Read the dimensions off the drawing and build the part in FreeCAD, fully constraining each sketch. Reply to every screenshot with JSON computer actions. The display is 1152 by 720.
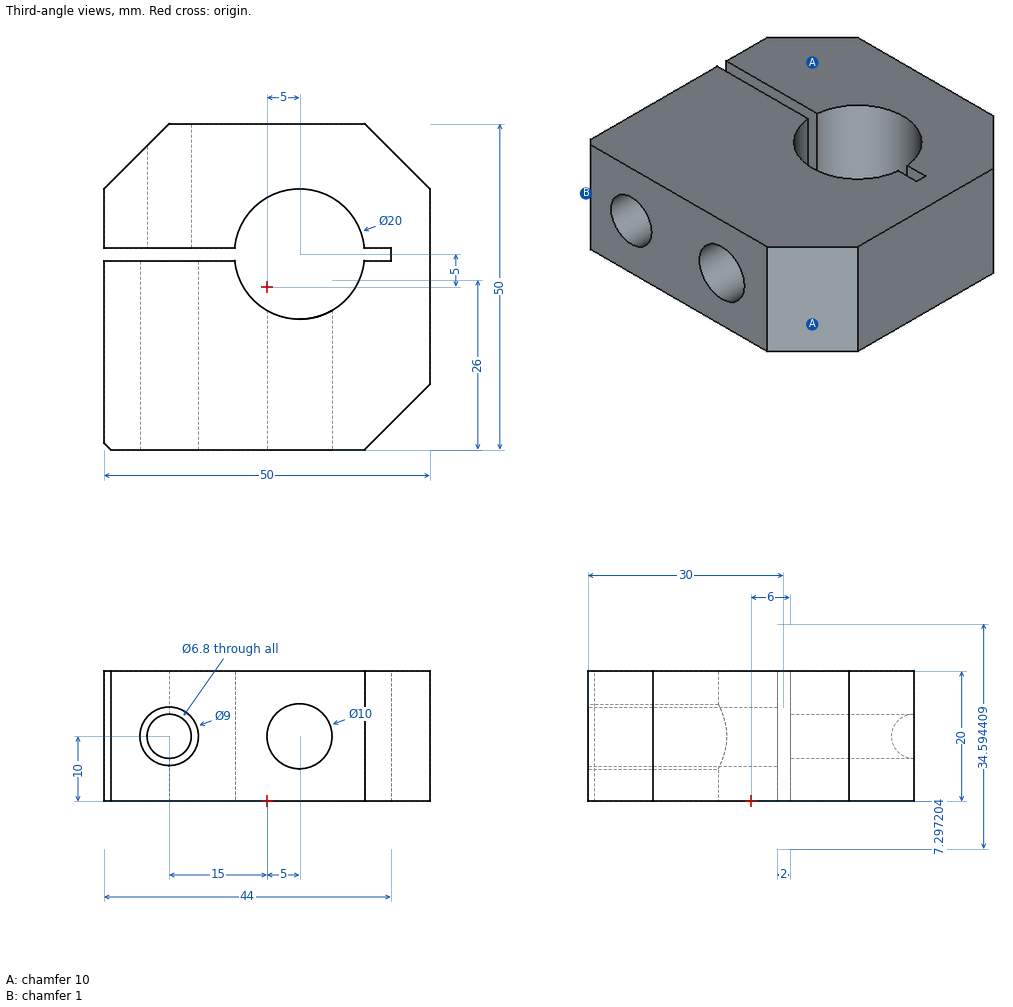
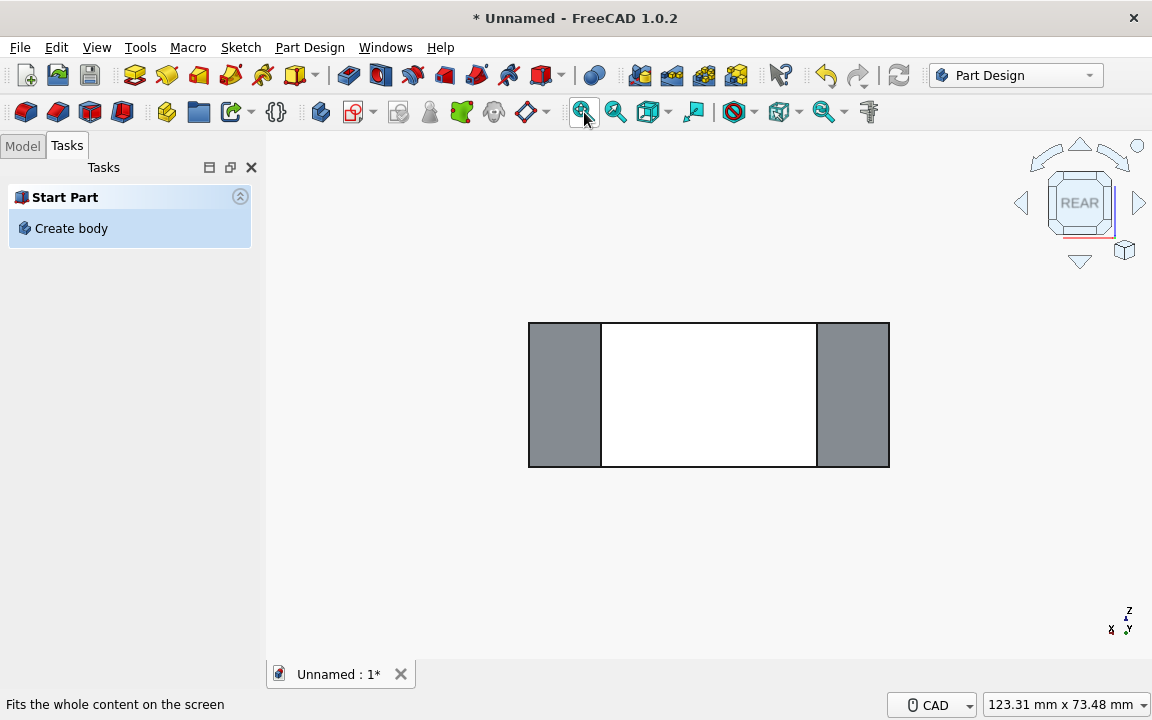
{"action": "key", "text": "0"}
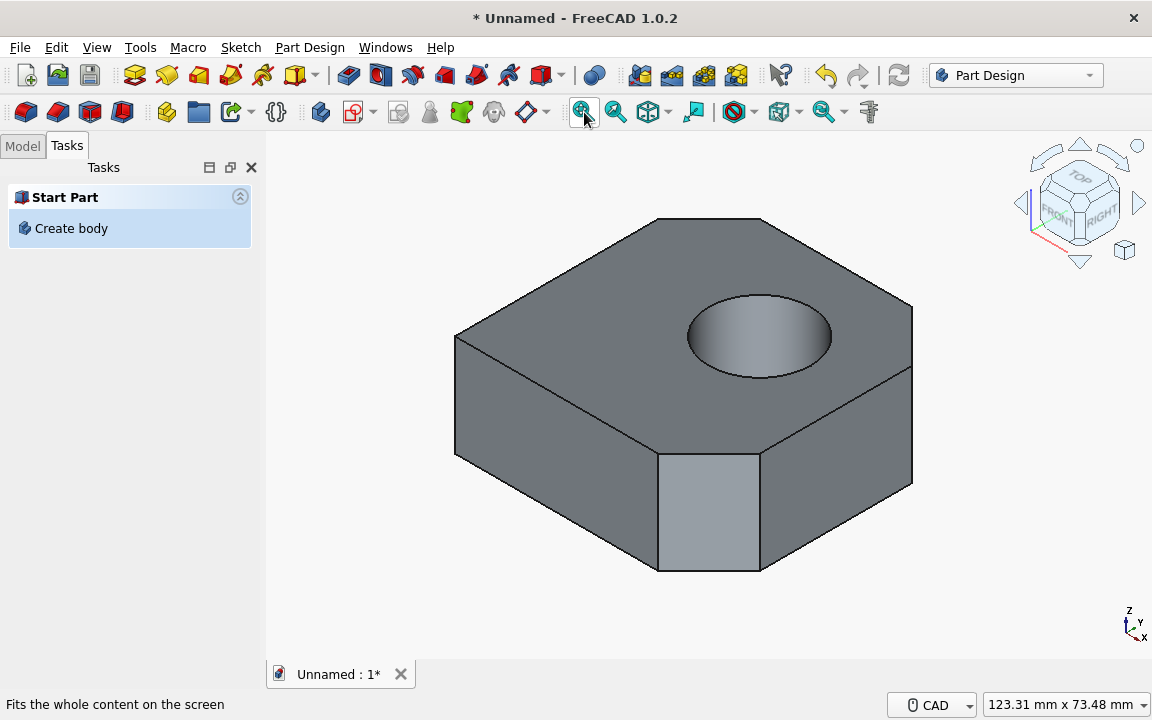
{"action": "key", "text": "2"}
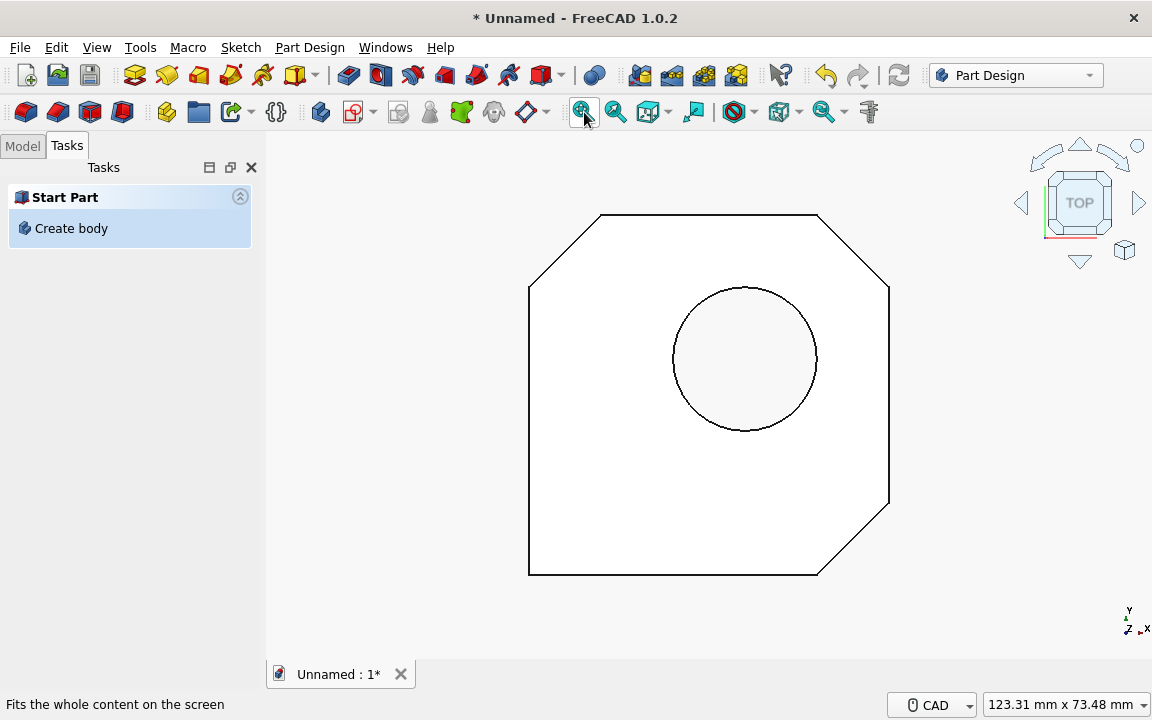
{"action": "key", "text": "1"}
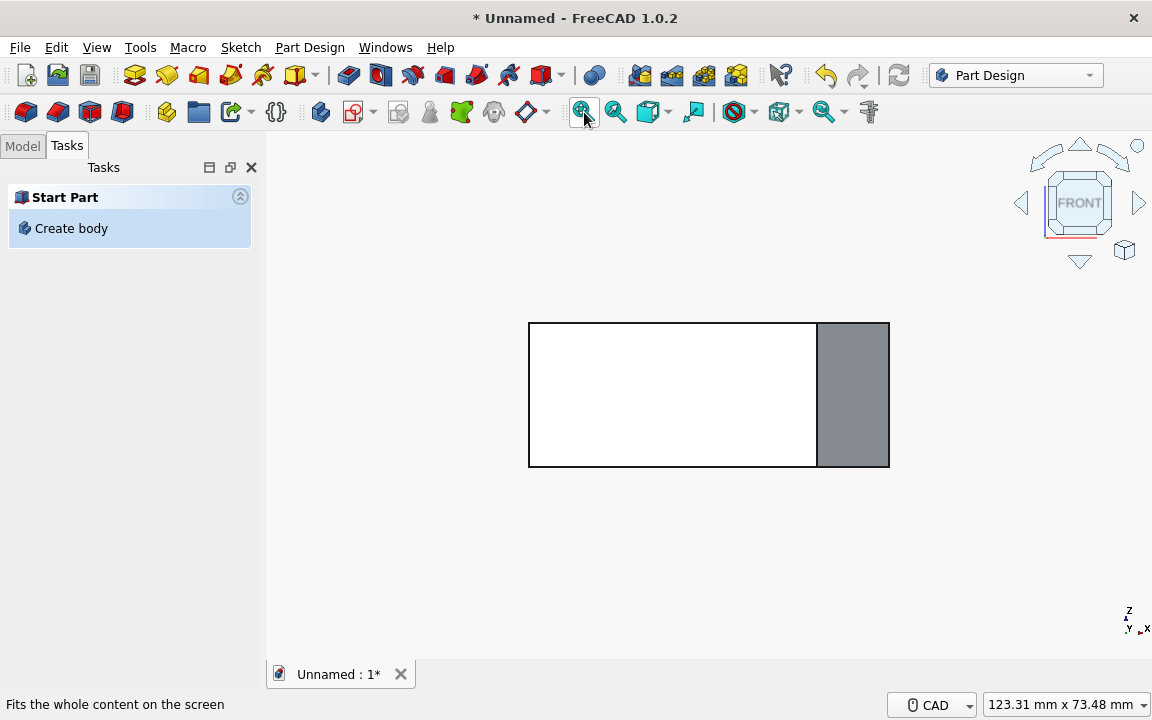
{"action": "left_click", "coordinate": [584, 112]}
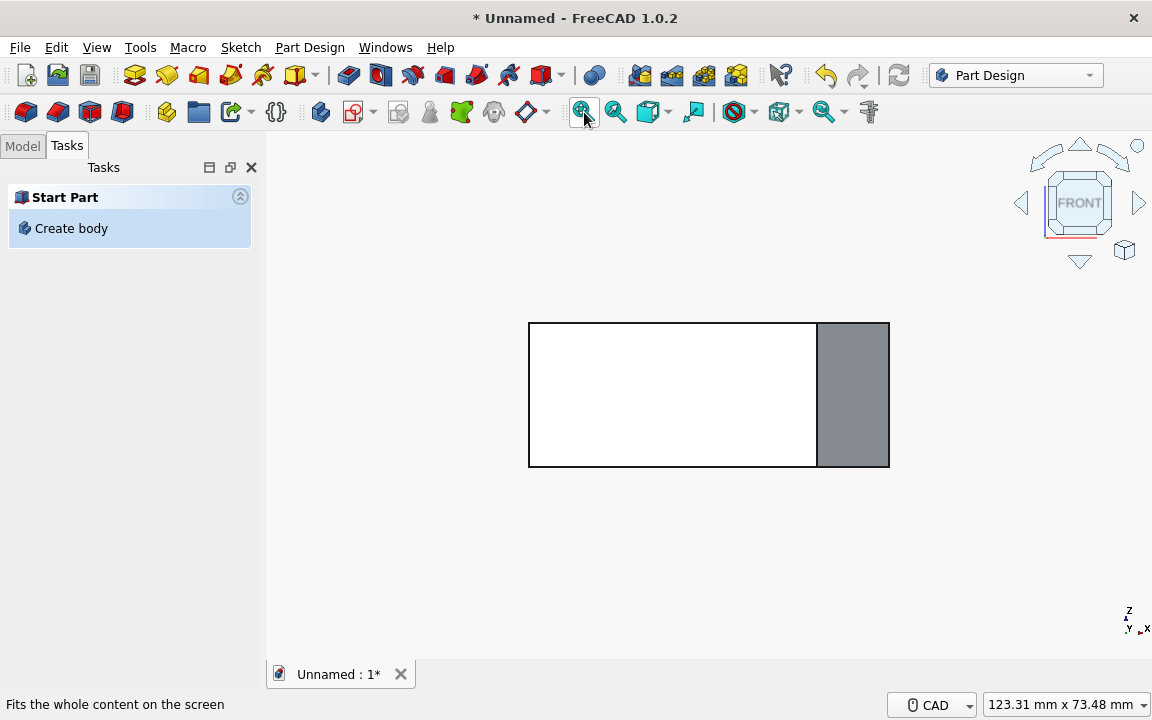
{"action": "left_click", "coordinate": [529, 394]}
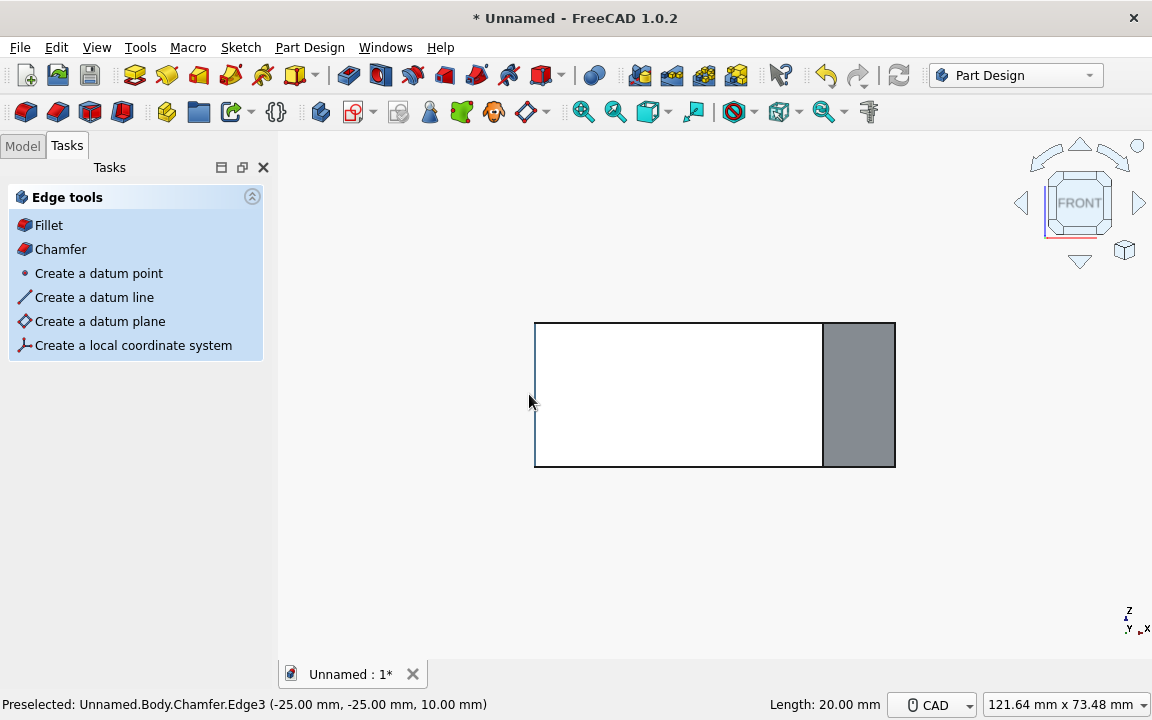
{"action": "left_click", "coordinate": [58, 112]}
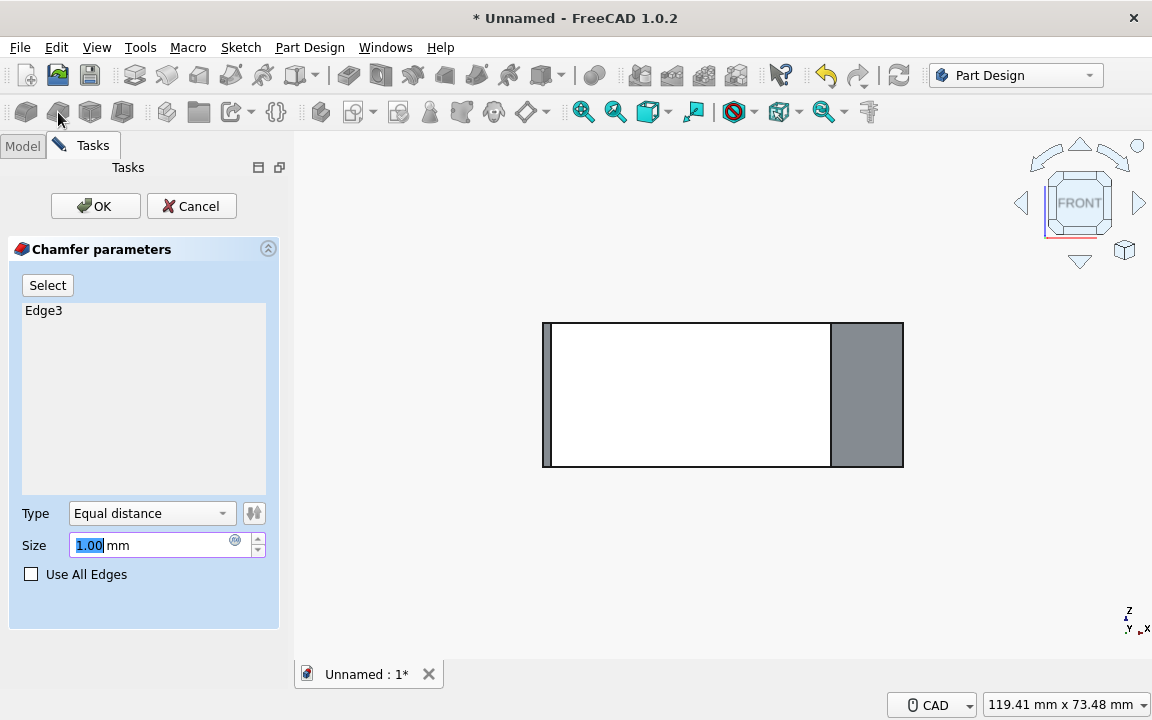
{"action": "type", "text": "1"}
{"action": "key", "text": "Tab"}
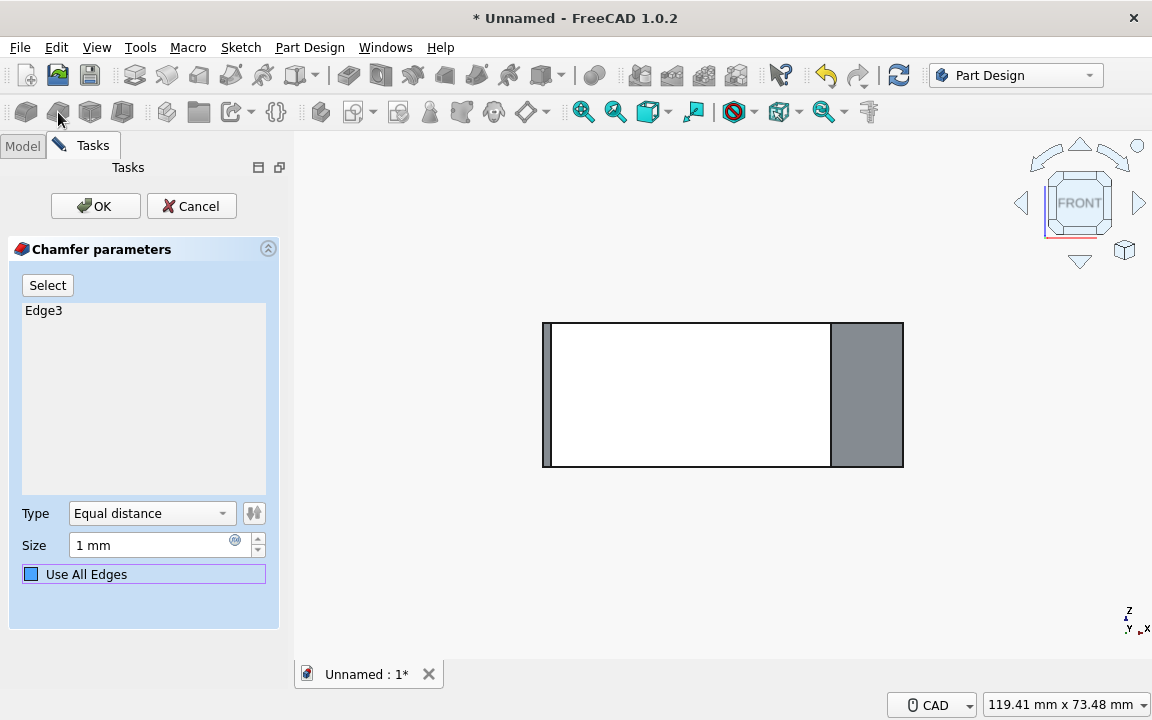
{"action": "left_click", "coordinate": [96, 206]}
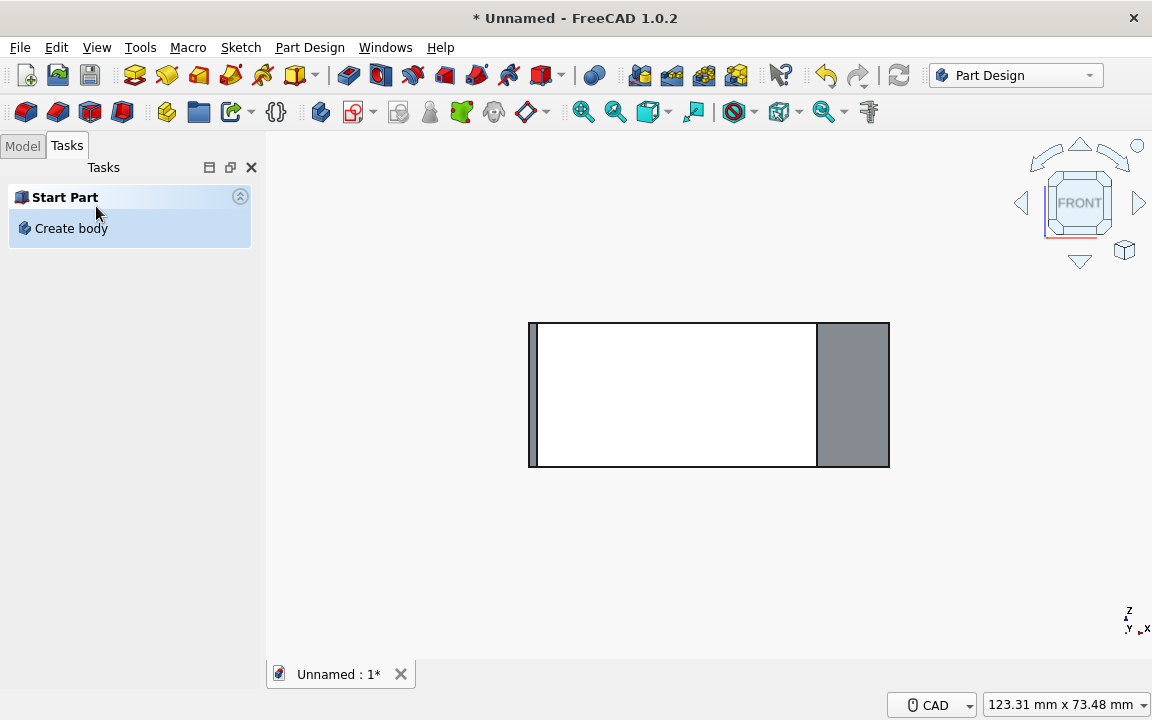
{"action": "left_click", "coordinate": [584, 112]}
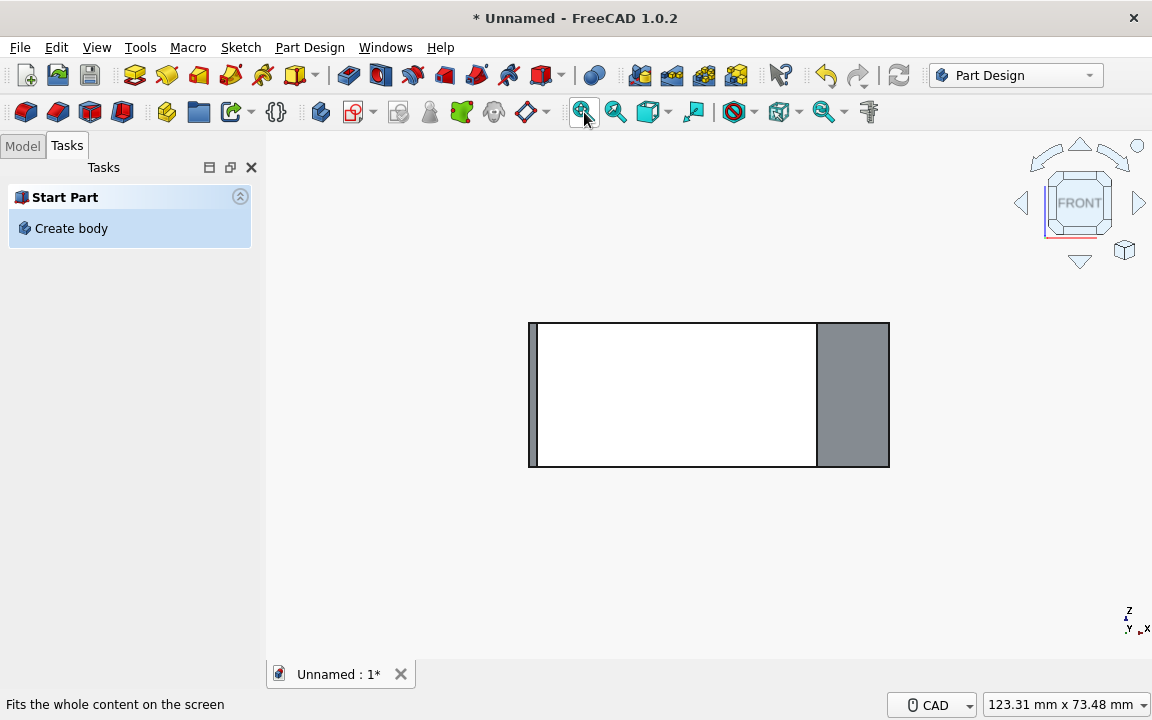
{"action": "key", "text": "4"}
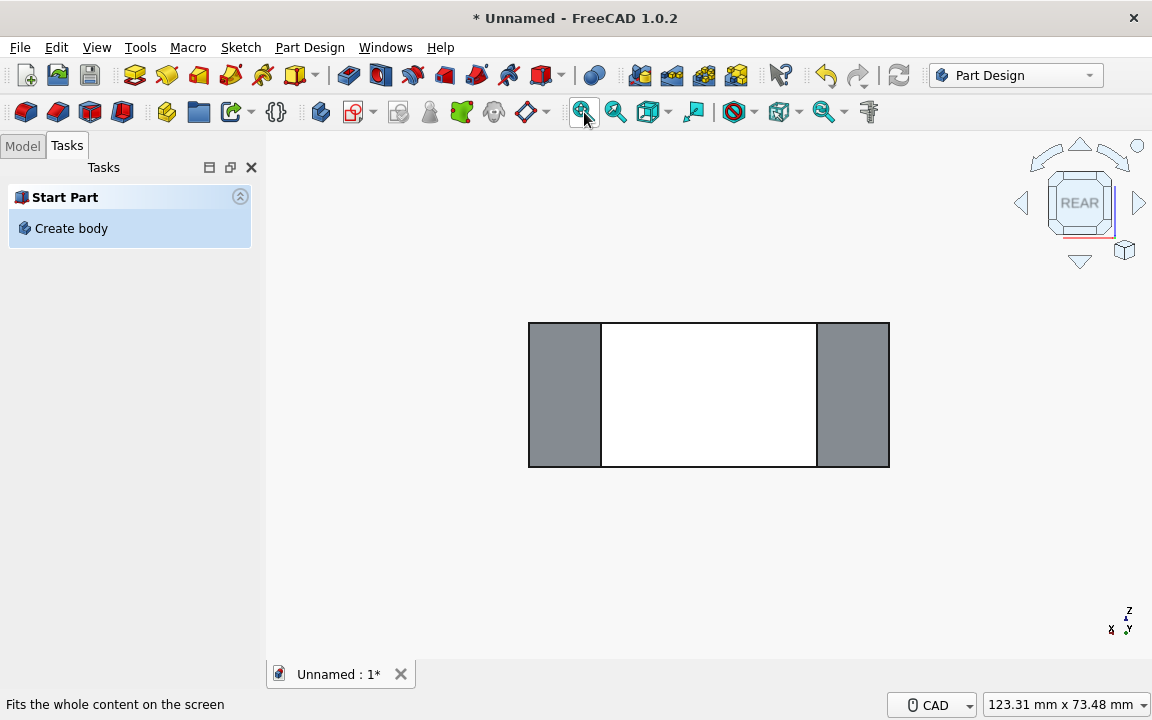
{"action": "left_click", "coordinate": [584, 112]}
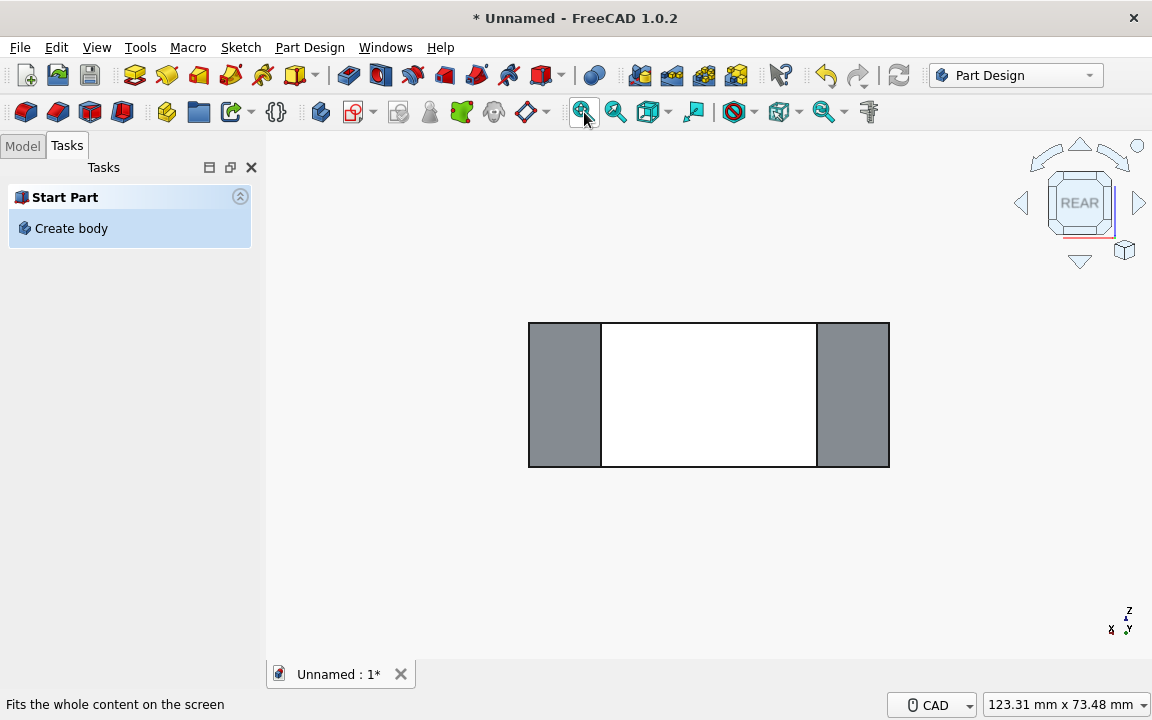
{"action": "left_click", "coordinate": [678, 394]}